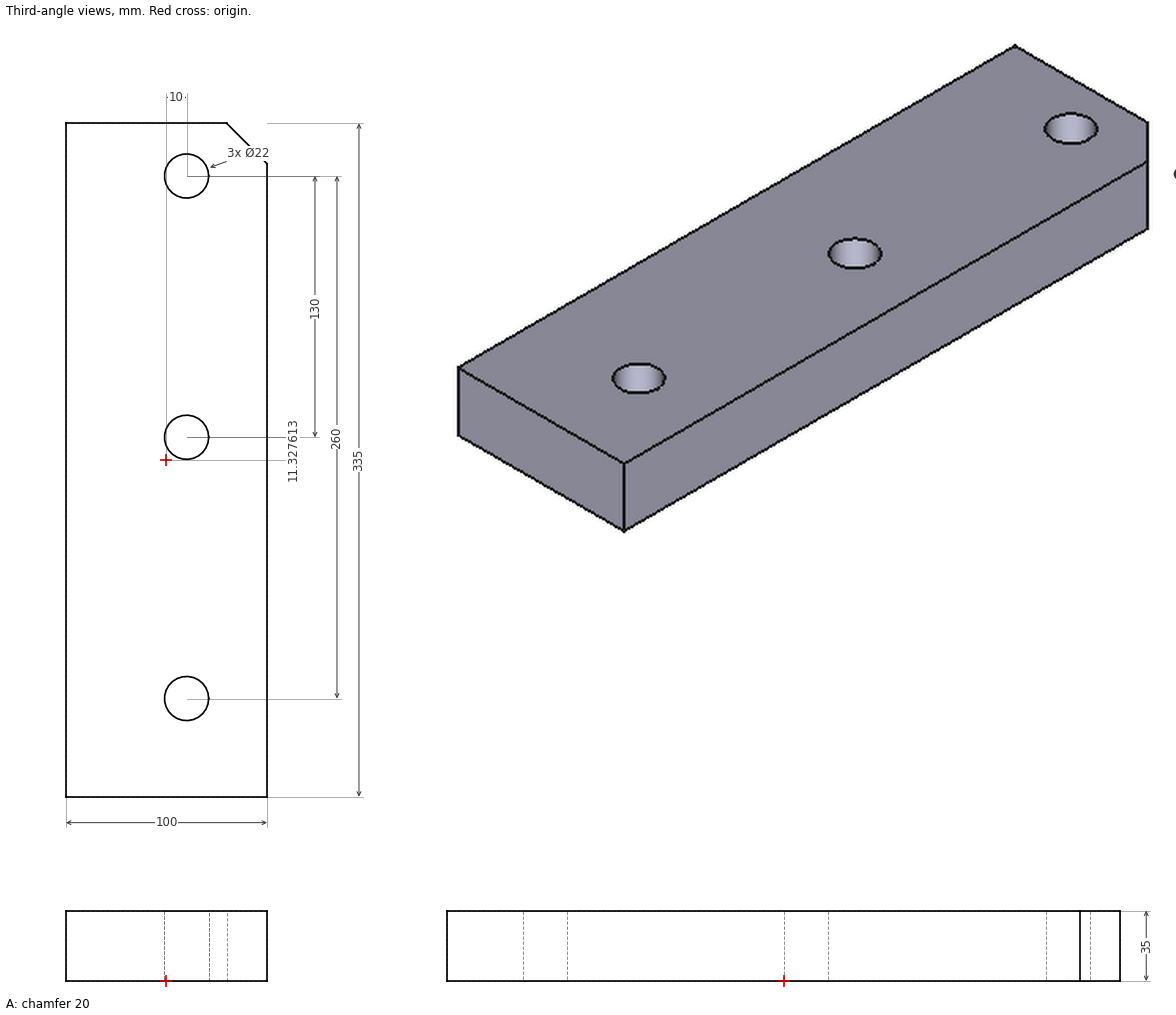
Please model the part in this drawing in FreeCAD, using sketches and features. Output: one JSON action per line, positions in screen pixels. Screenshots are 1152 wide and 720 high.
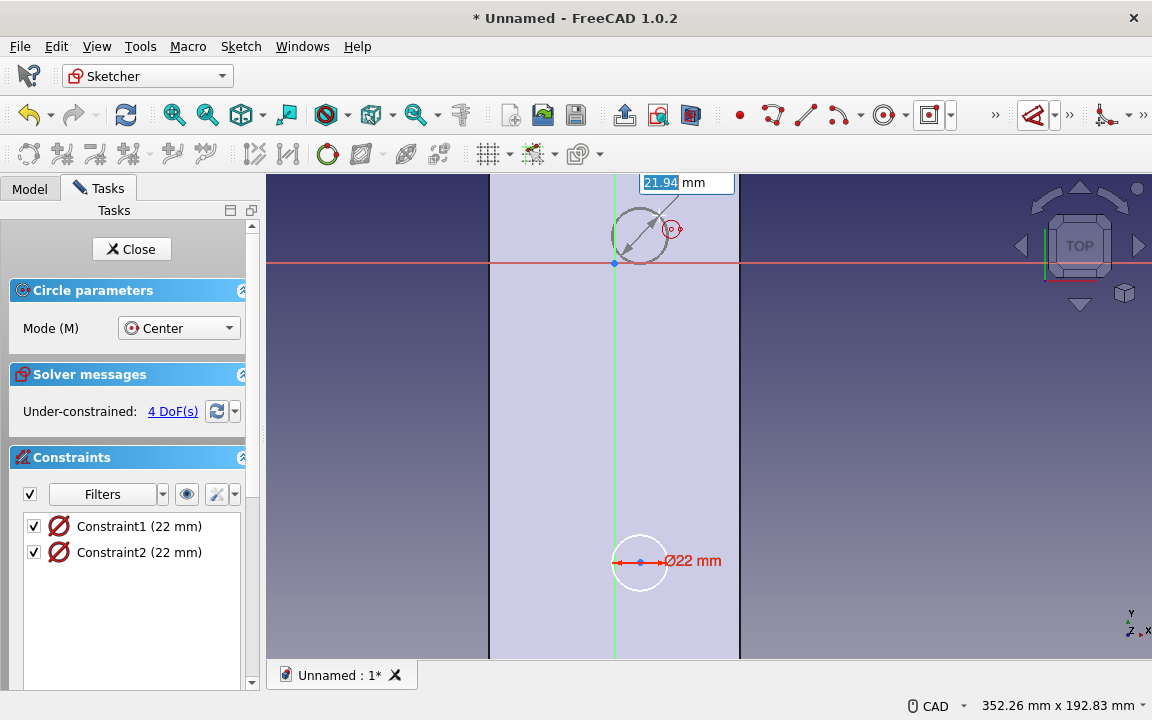
{"action": "type", "text": "22"}
{"action": "key", "text": "Return"}
{"action": "key", "text": "Escape"}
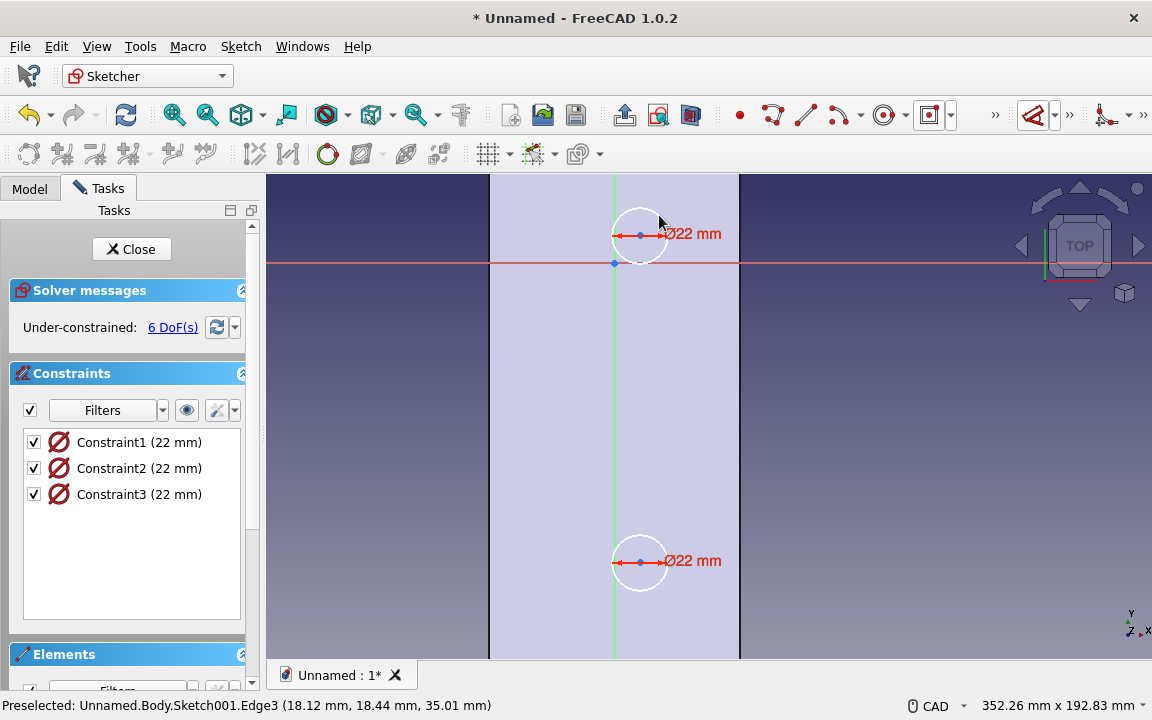
{"action": "scroll", "coordinate": [641, 565], "scroll_direction": "down", "scroll_amount": 4}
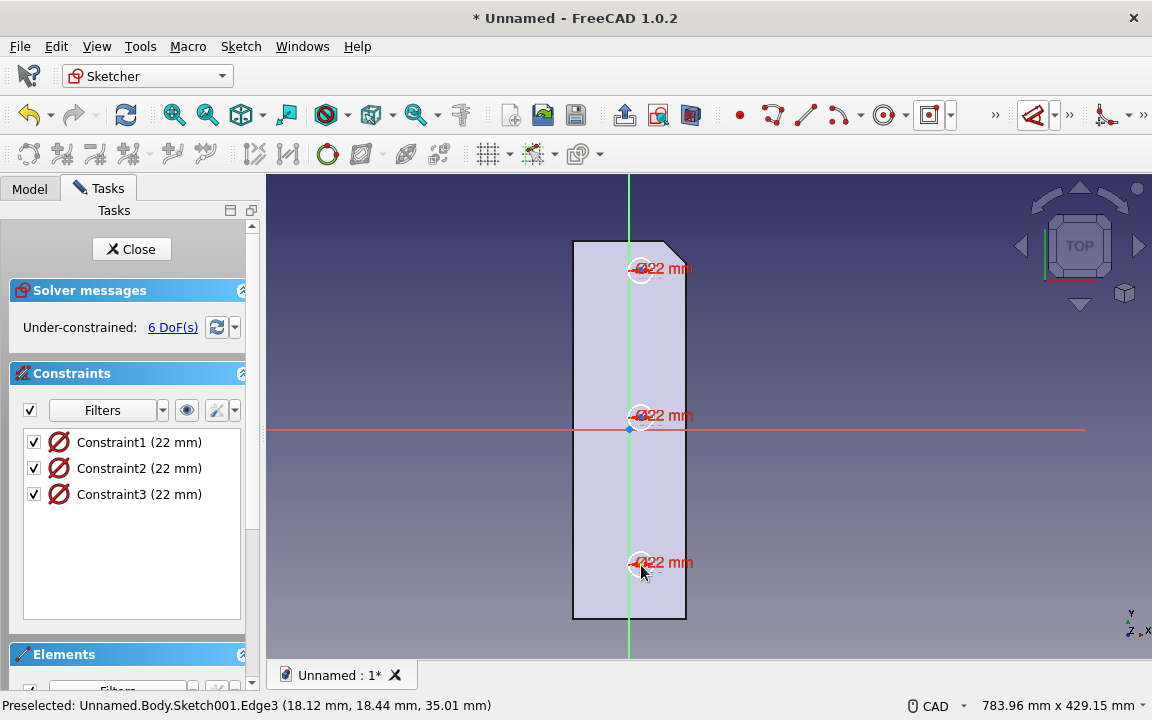
{"action": "left_click", "coordinate": [641, 271]}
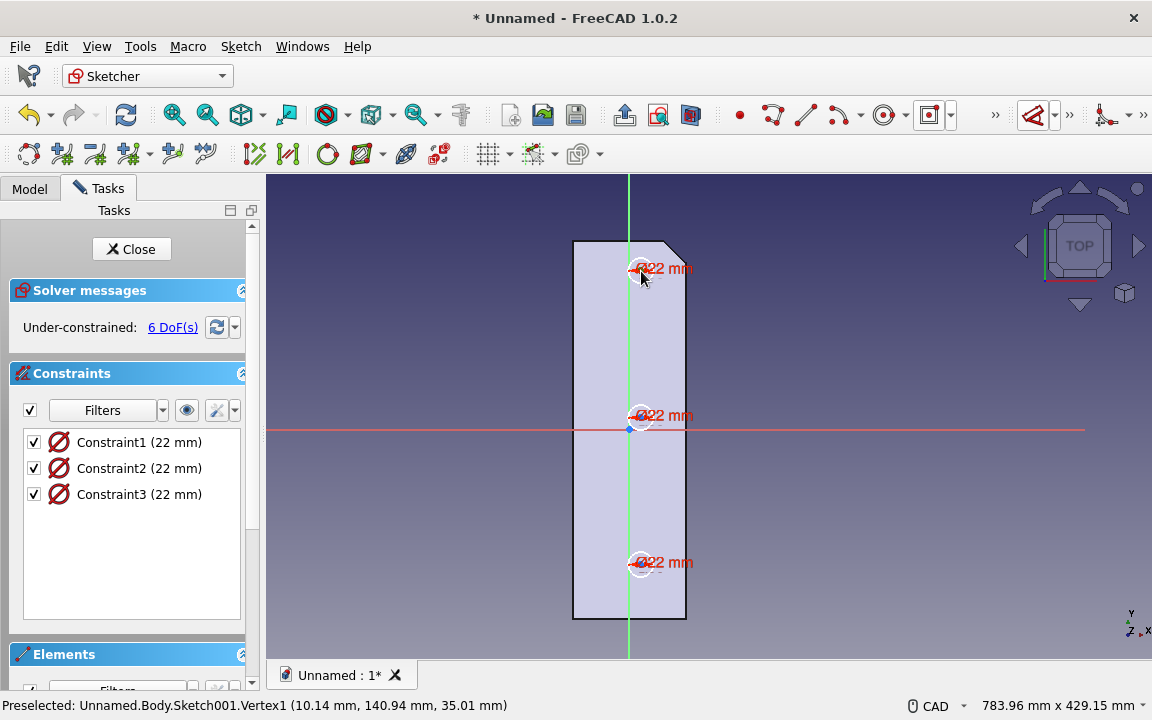
{"action": "left_click", "coordinate": [641, 565]}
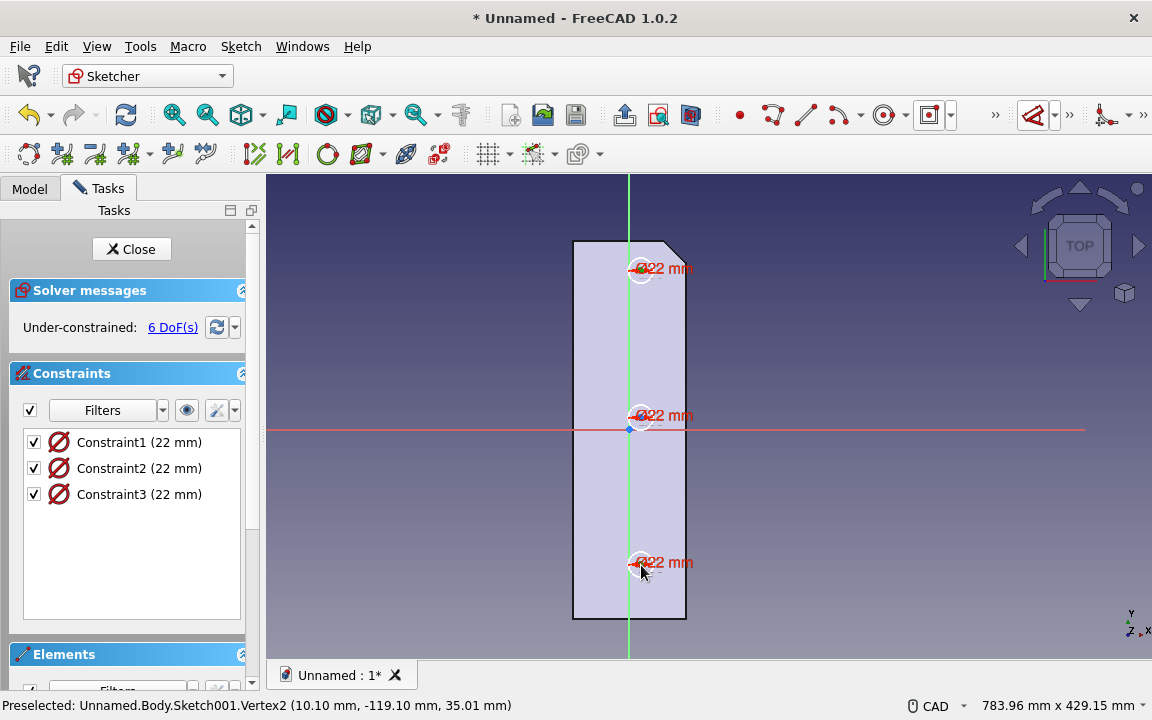
{"action": "key", "text": "v"}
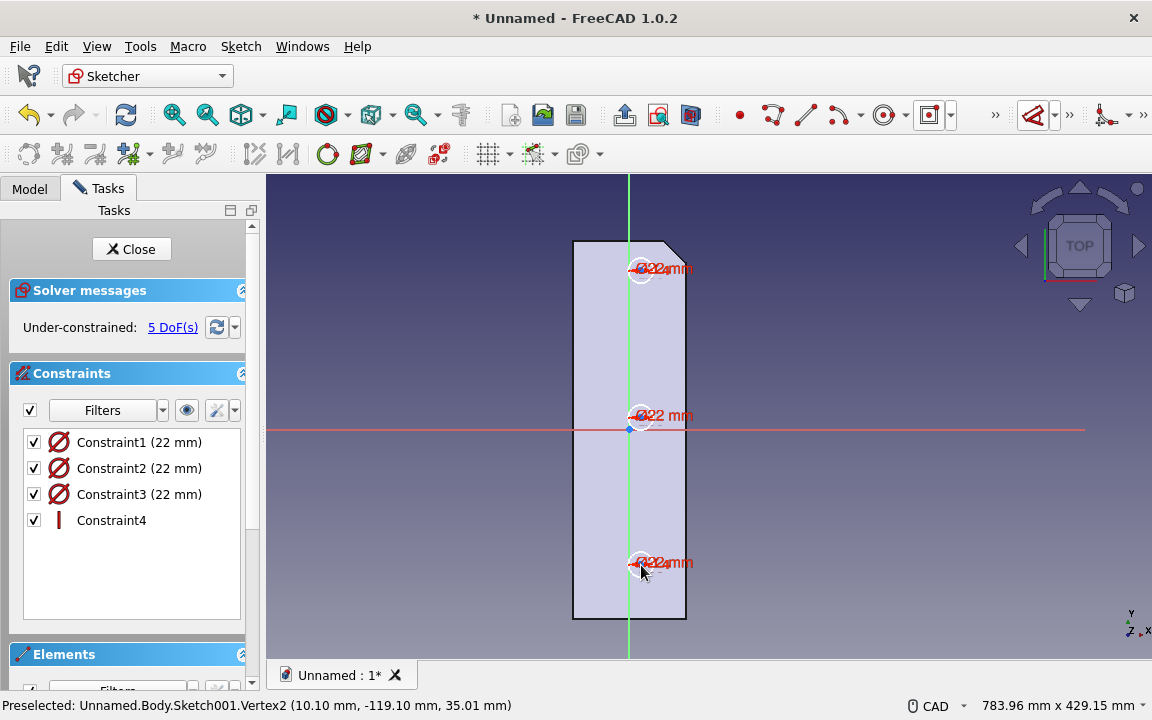
{"action": "left_click", "coordinate": [641, 271]}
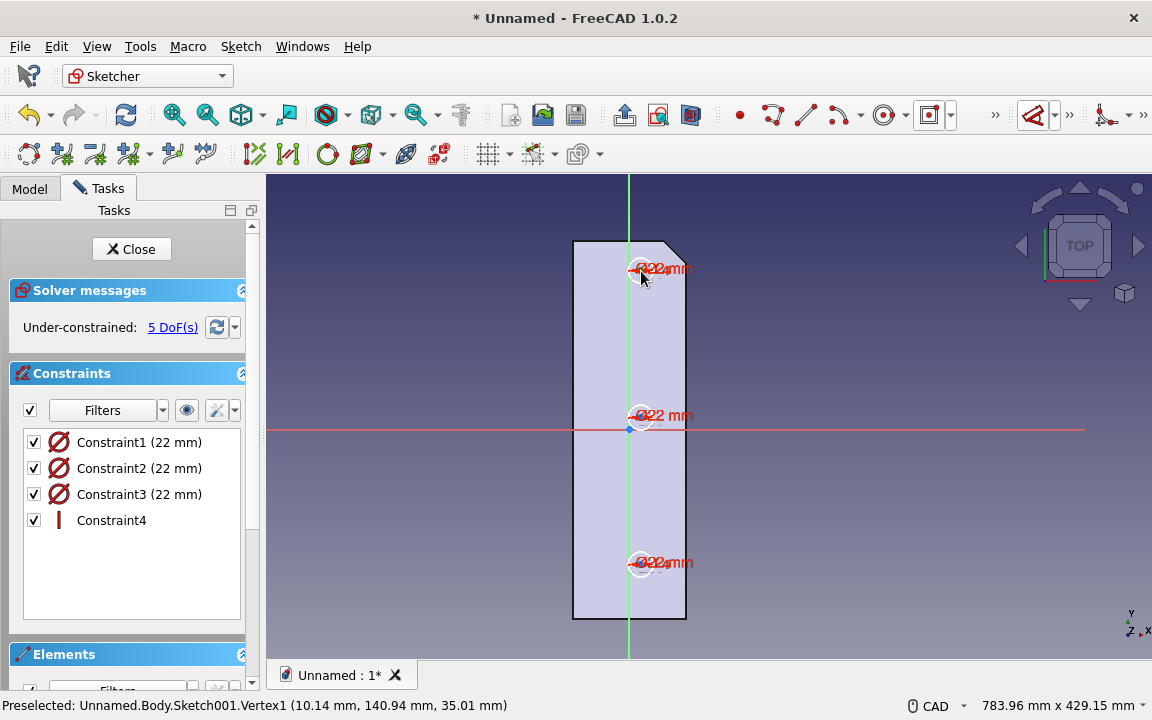
{"action": "left_click", "coordinate": [641, 418]}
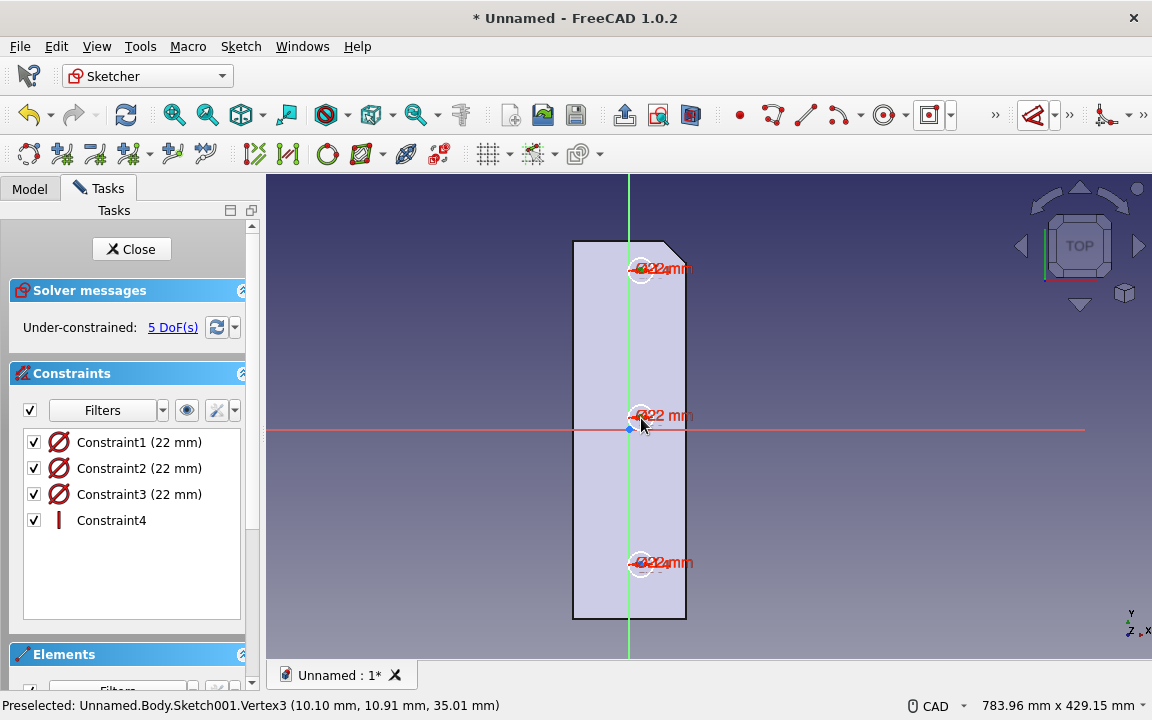
{"action": "key", "text": "v"}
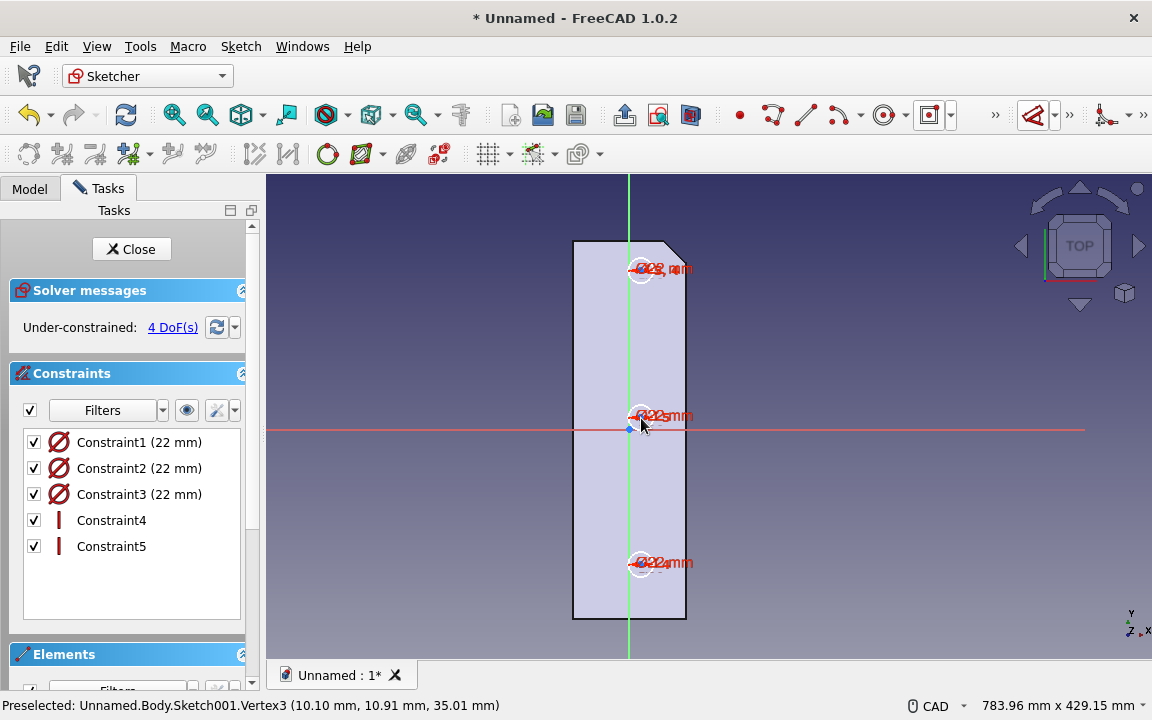
{"action": "left_click", "coordinate": [1032, 116]}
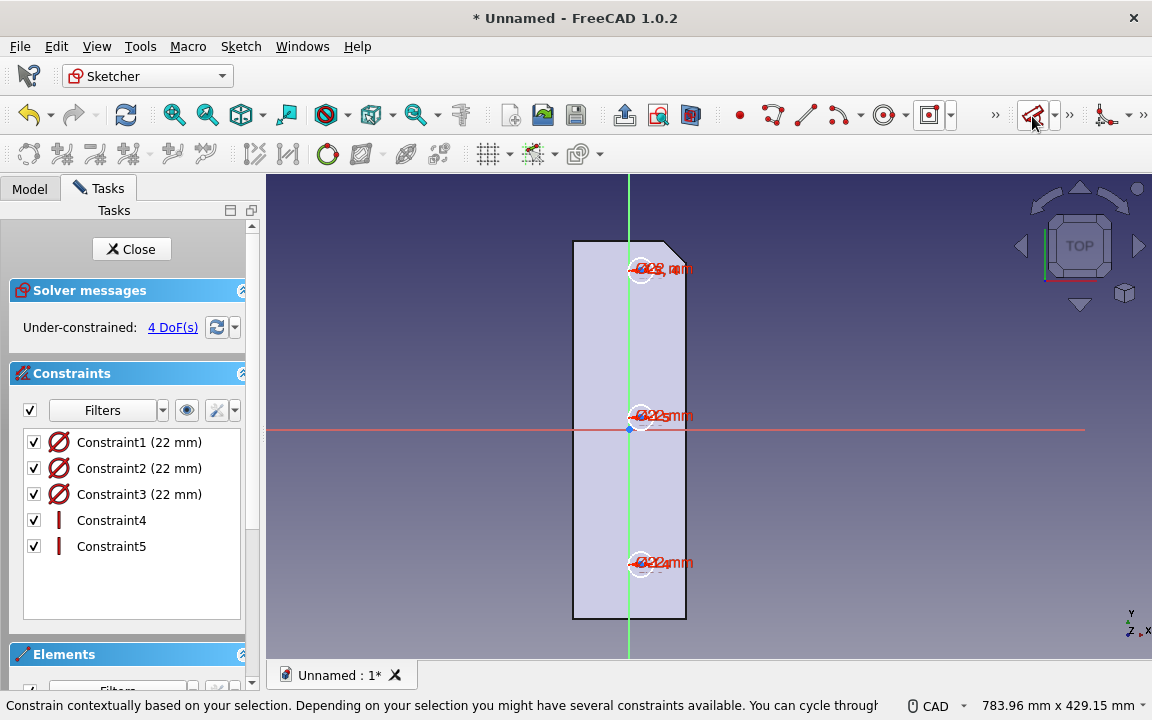
{"action": "scroll", "coordinate": [641, 271], "scroll_direction": "up", "scroll_amount": 7}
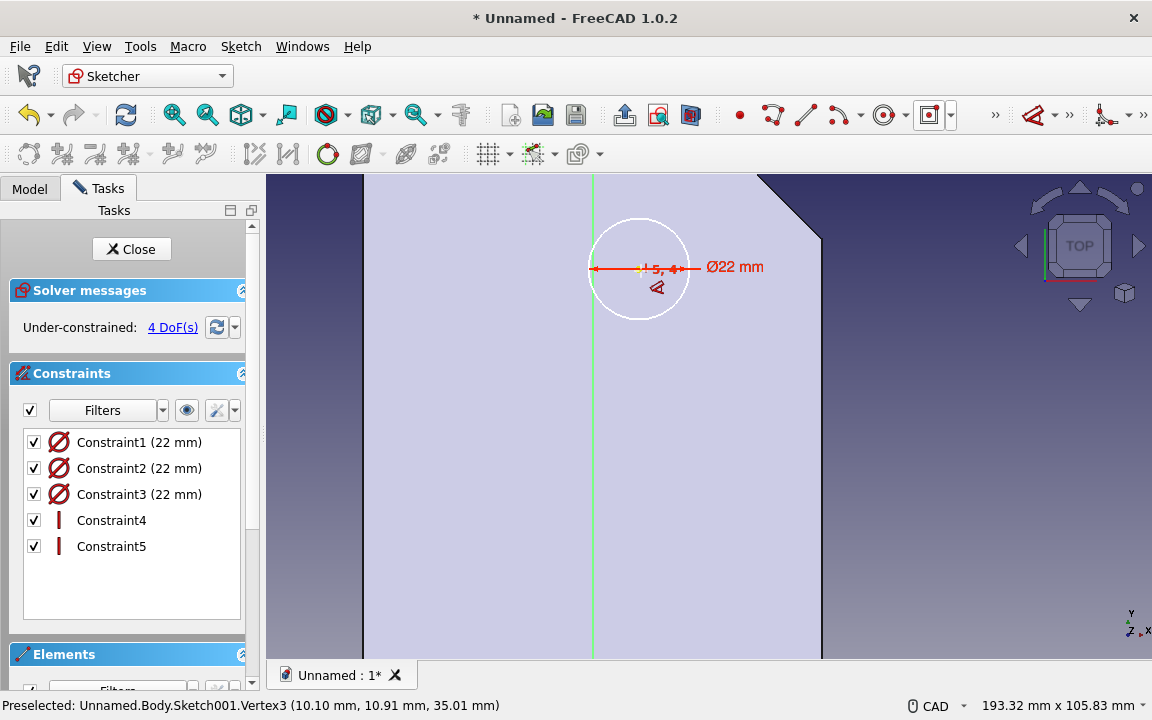
{"action": "left_click", "coordinate": [639, 269]}
{"action": "left_click", "coordinate": [626, 235]}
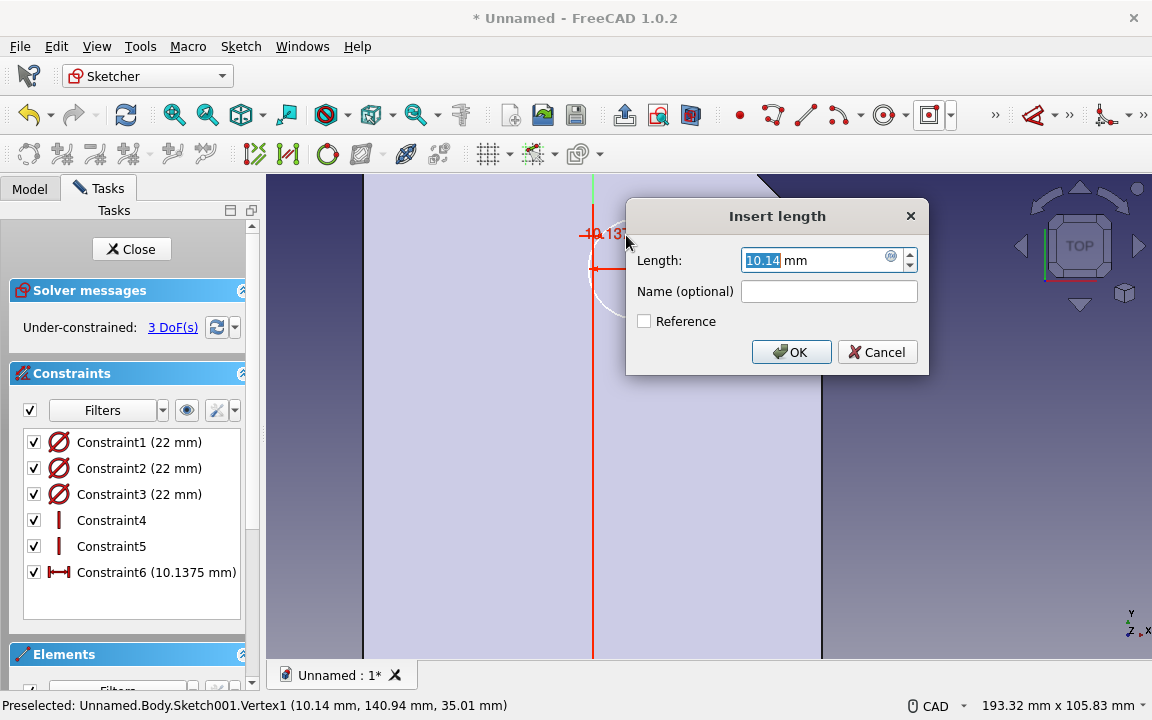
{"action": "type", "text": "10"}
{"action": "key", "text": "Return"}